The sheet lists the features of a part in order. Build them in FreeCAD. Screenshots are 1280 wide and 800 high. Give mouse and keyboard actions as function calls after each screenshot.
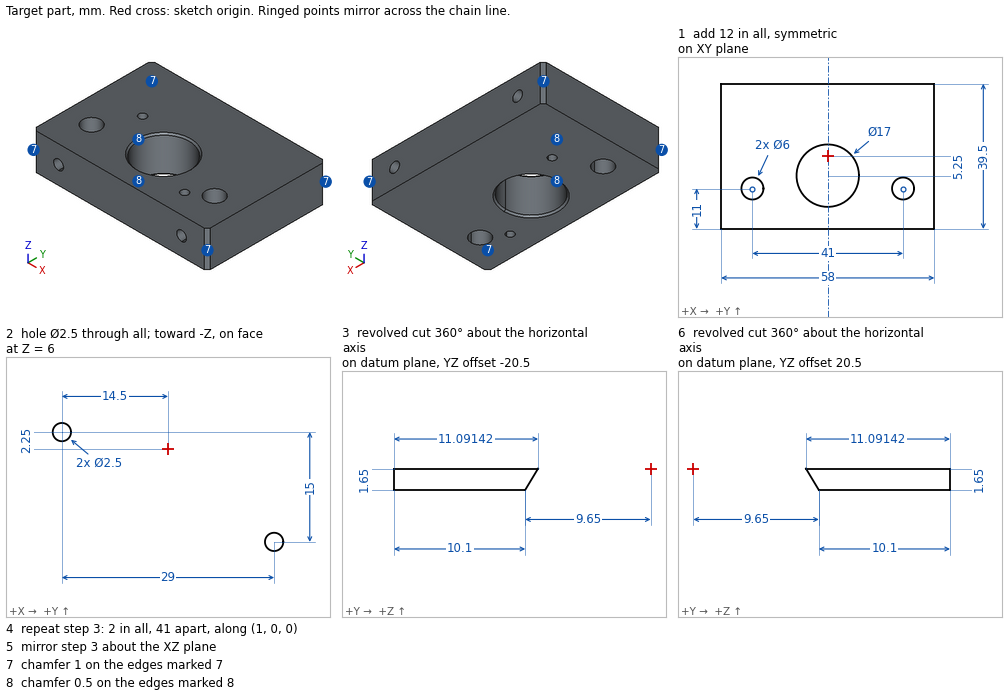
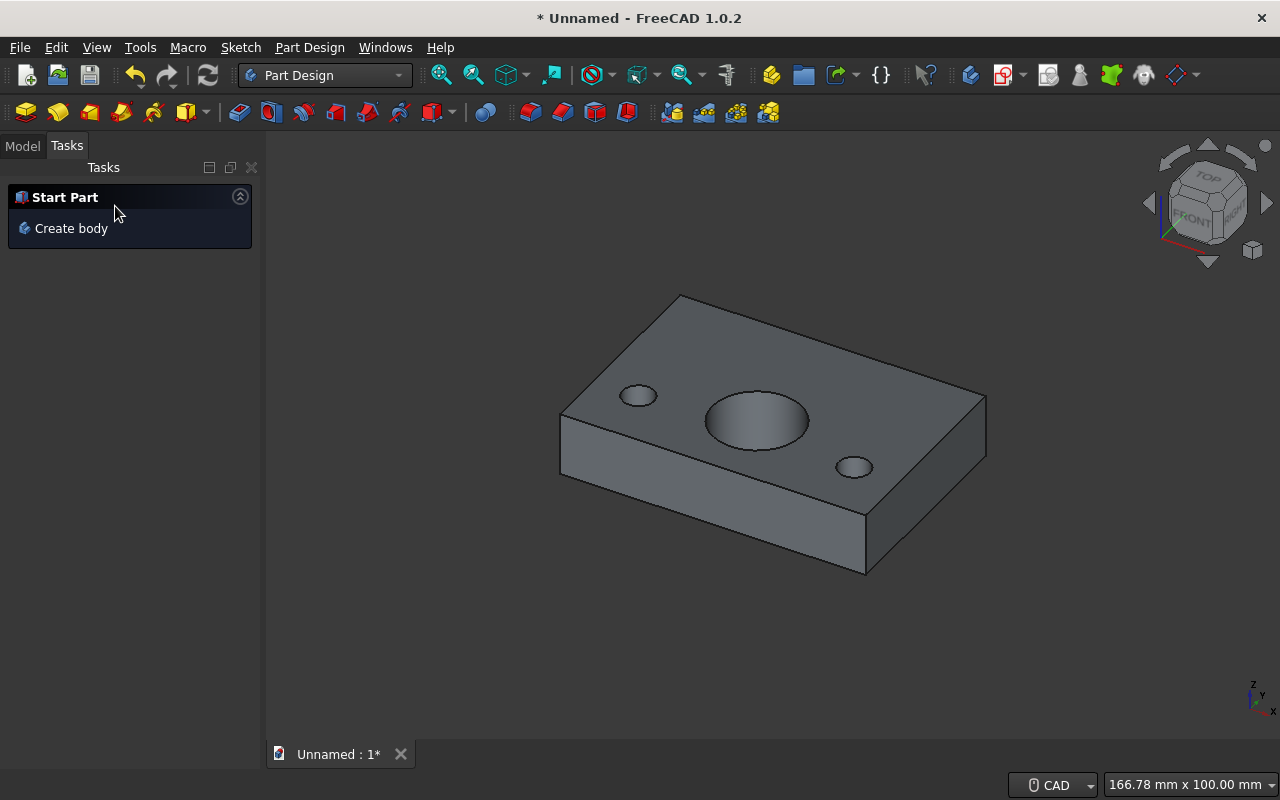
click(877, 416)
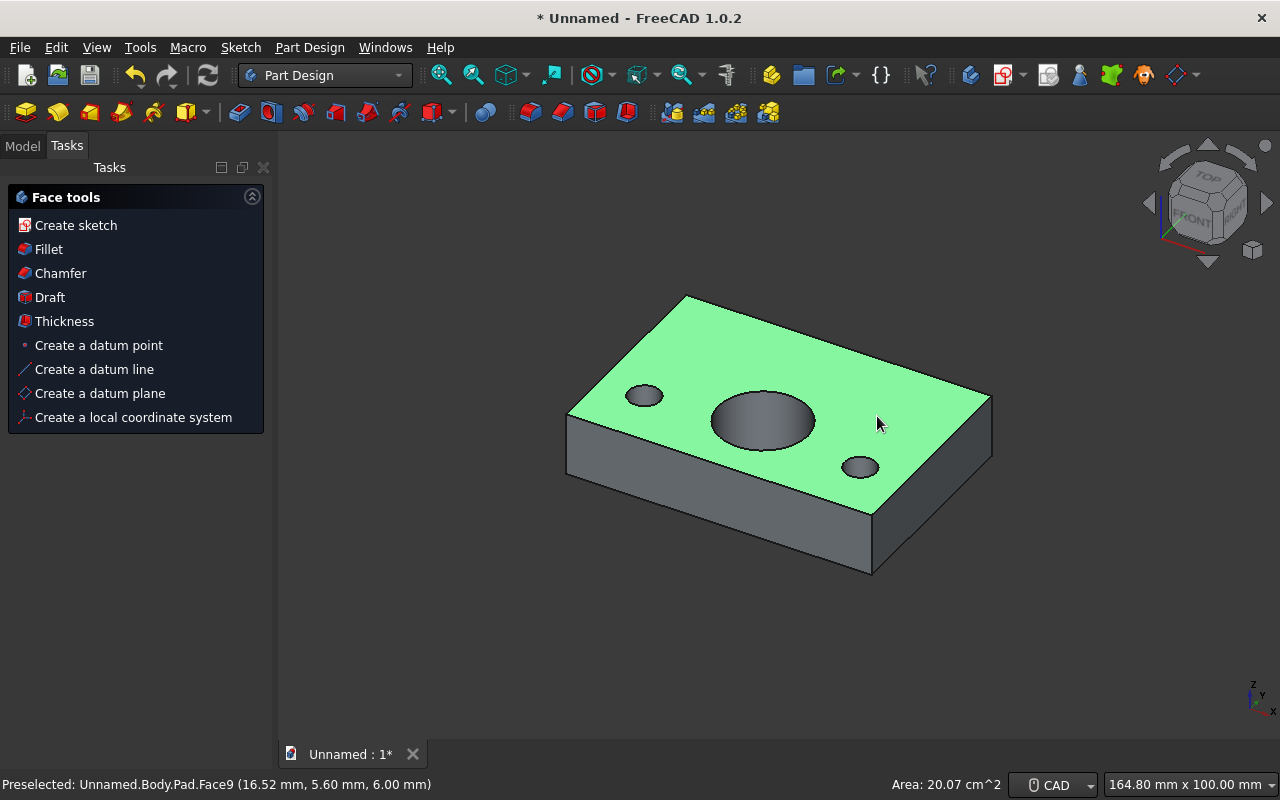
click(1004, 76)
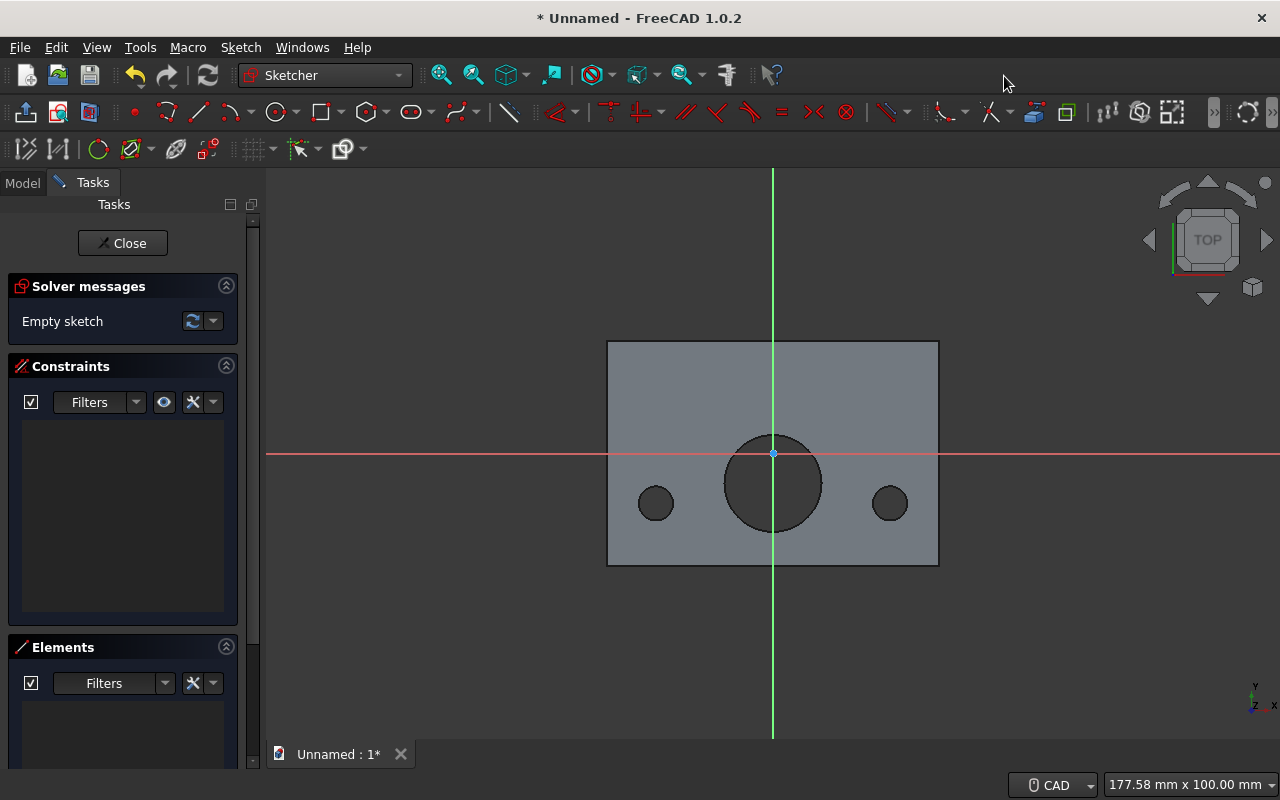
scroll(803, 496, up, 6)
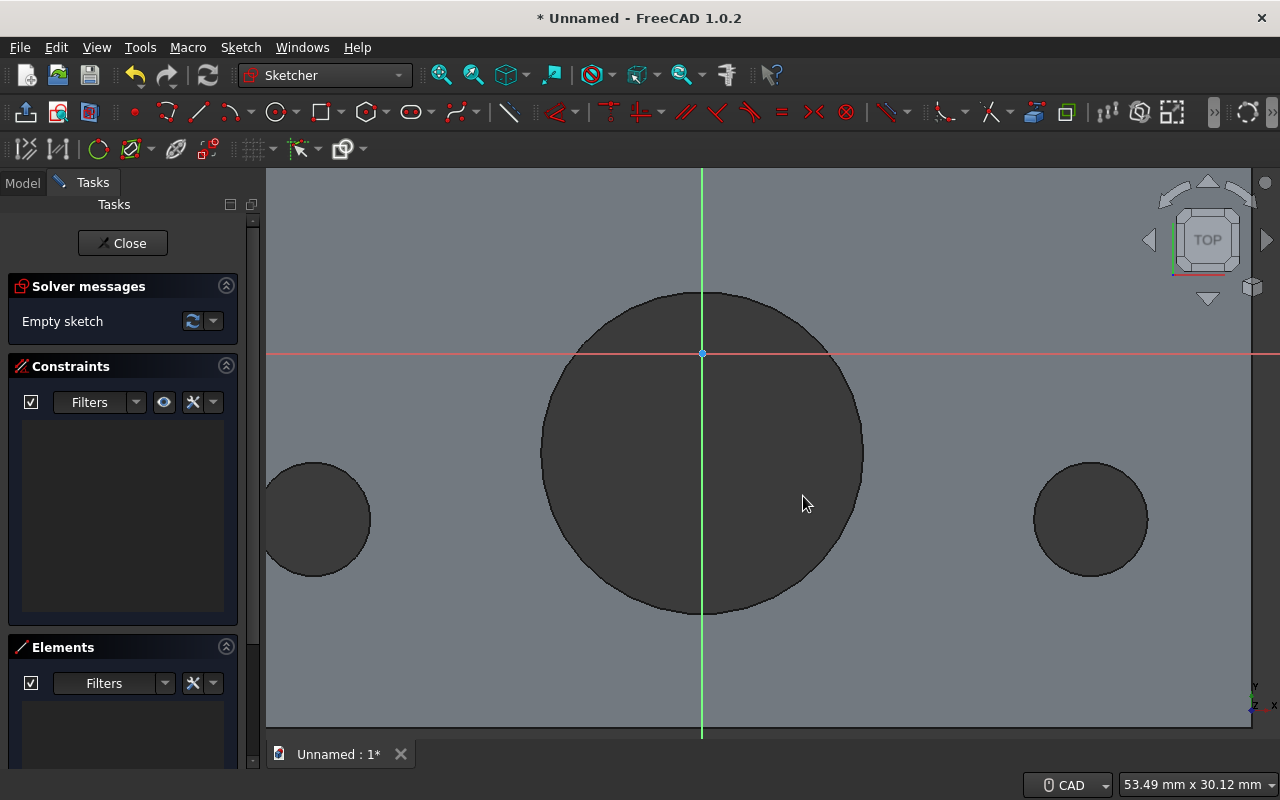
click(276, 112)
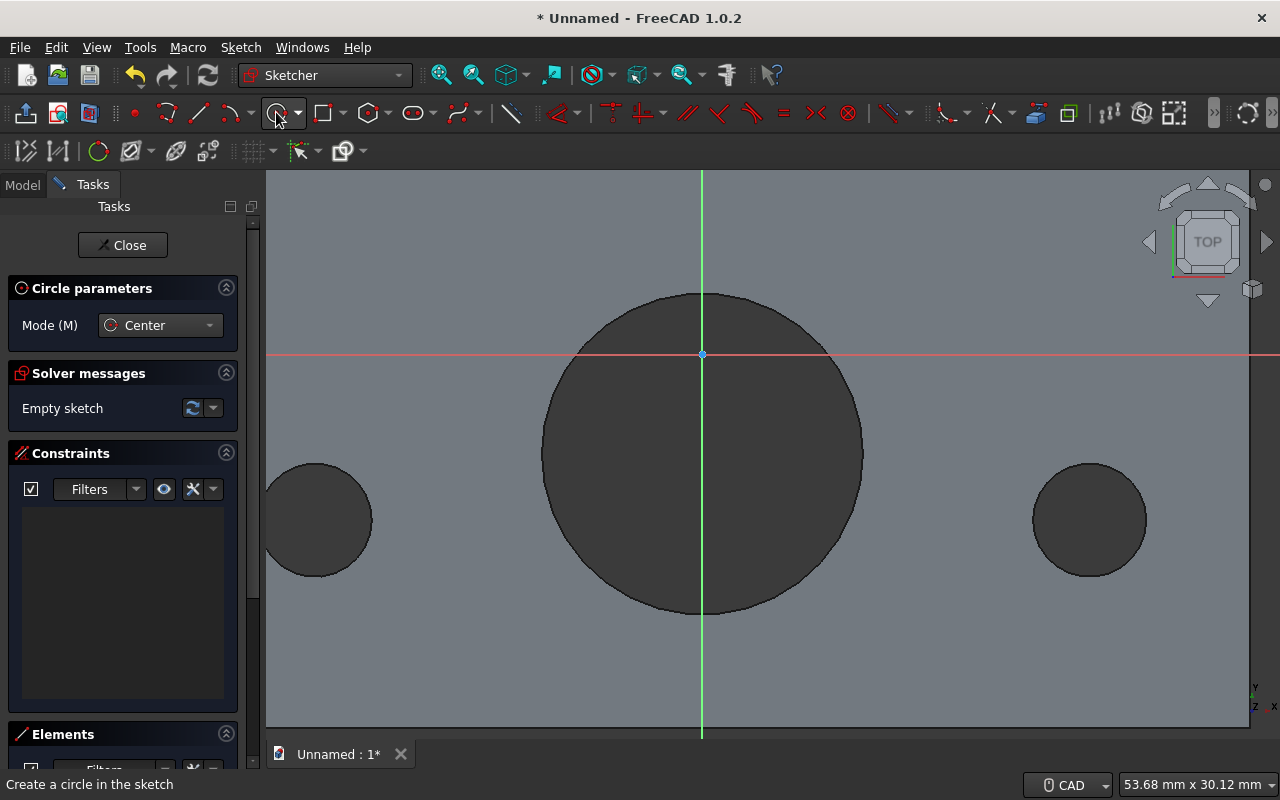
click(428, 312)
click(445, 296)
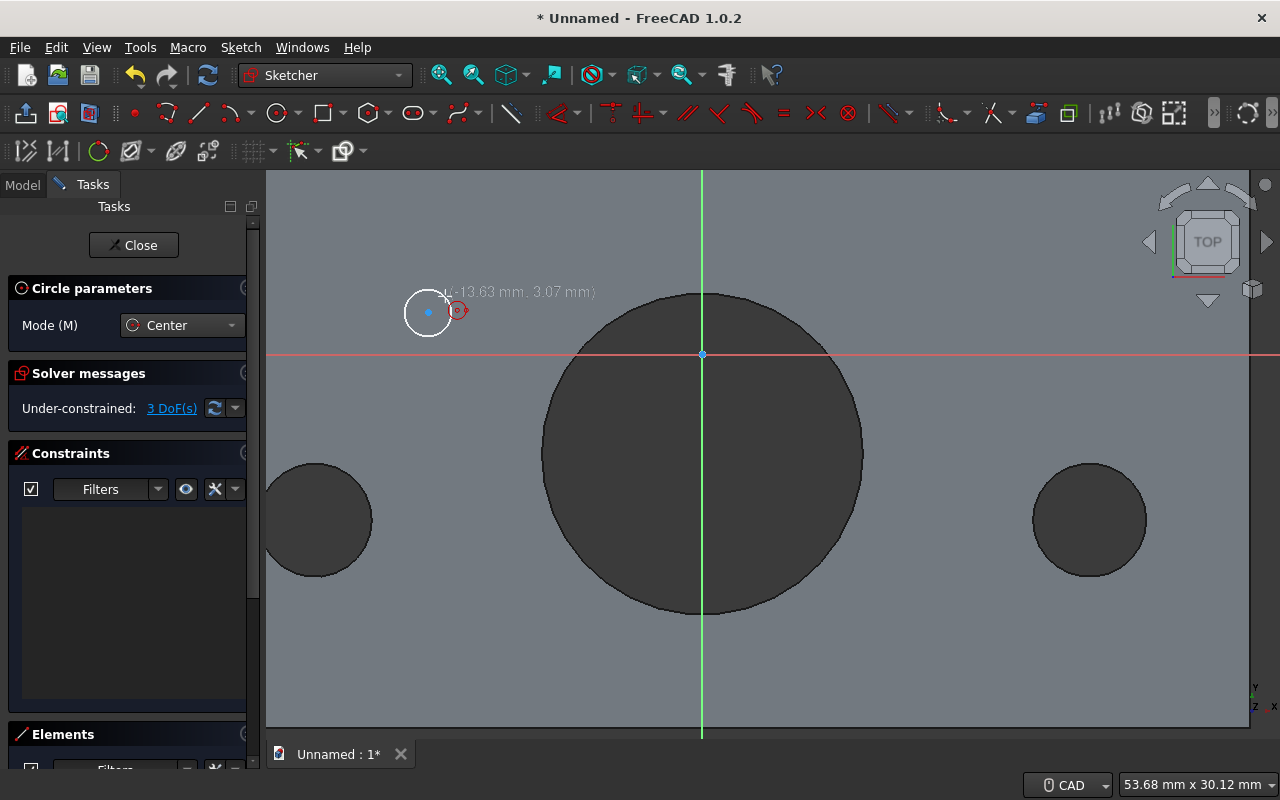
click(976, 596)
click(993, 579)
key(Escape)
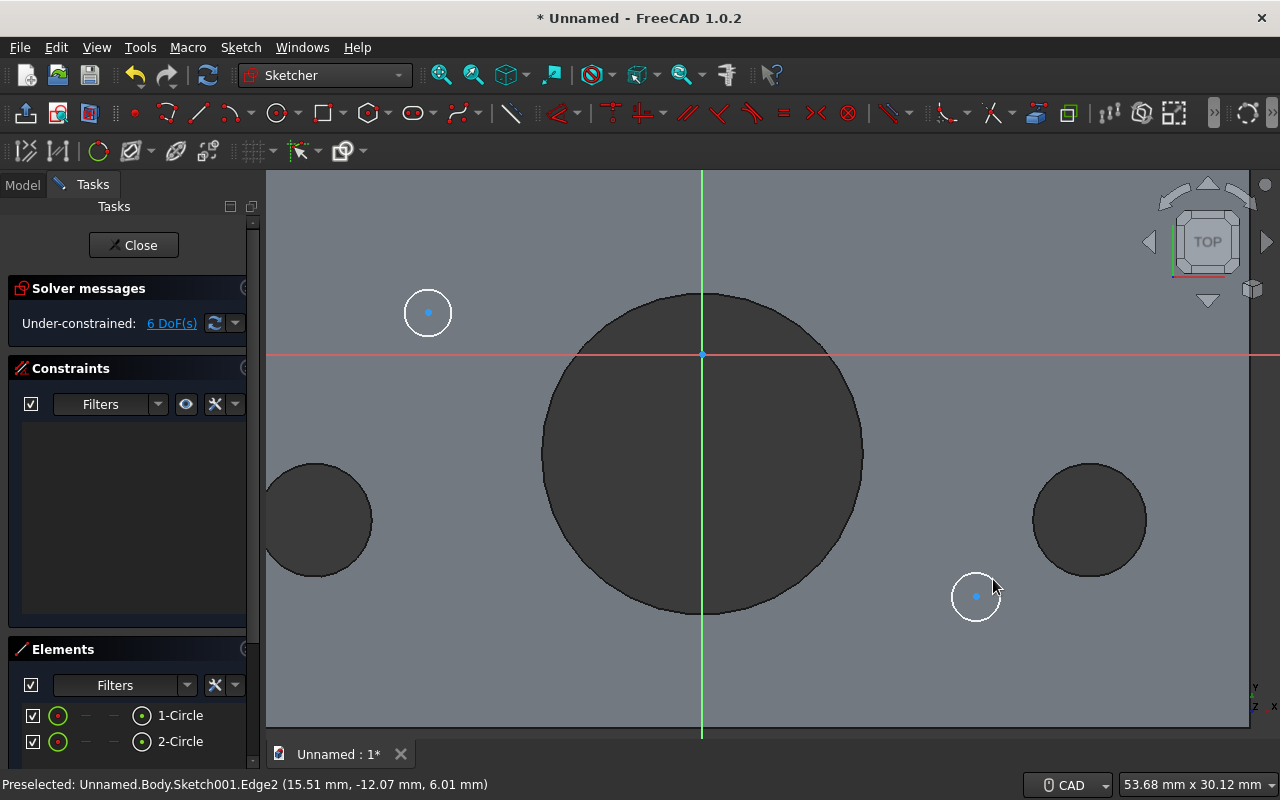
click(444, 296)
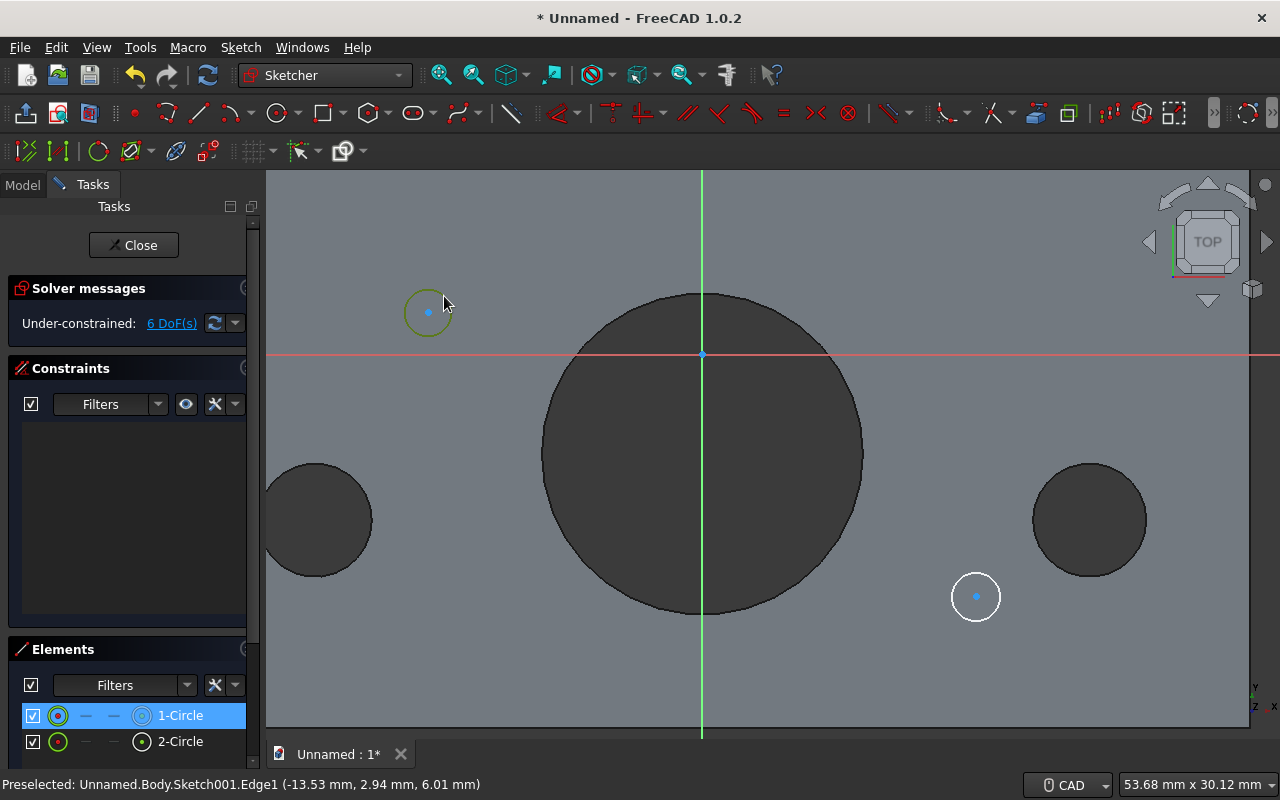
click(993, 580)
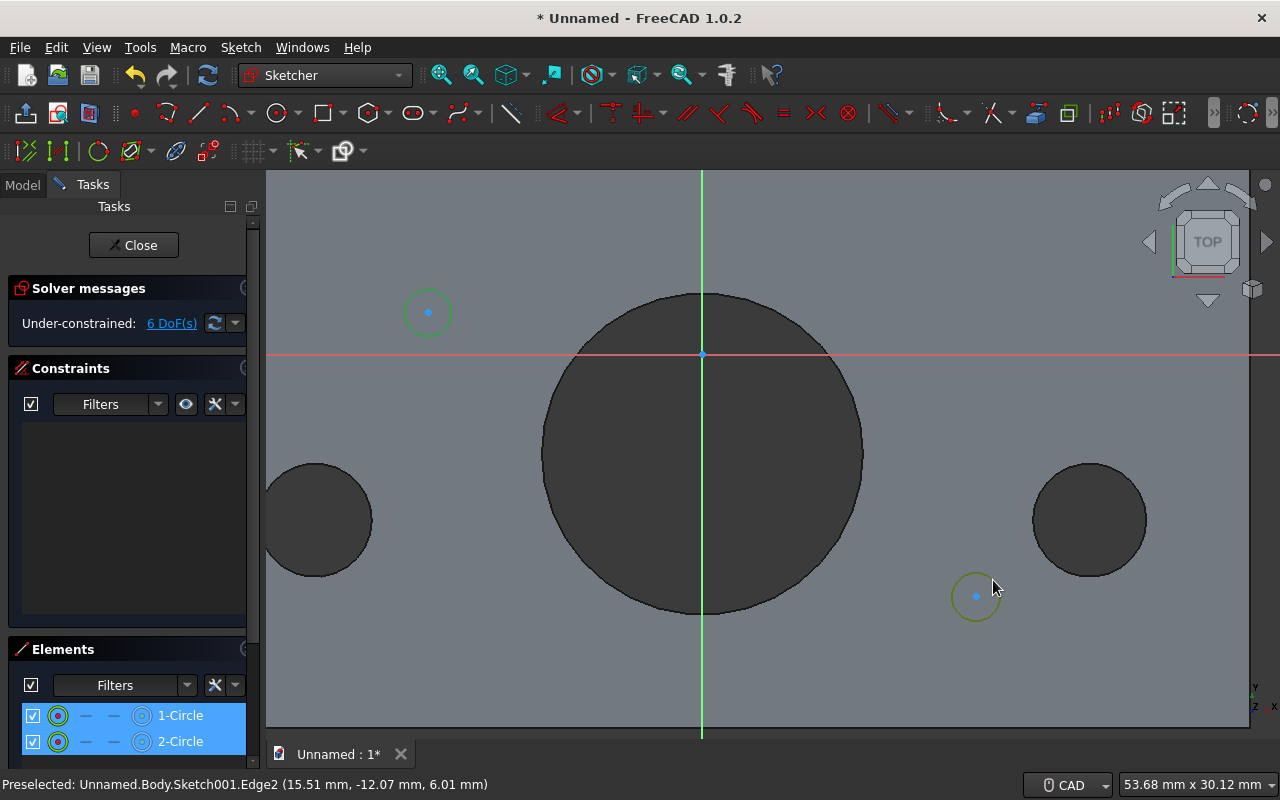
key(e)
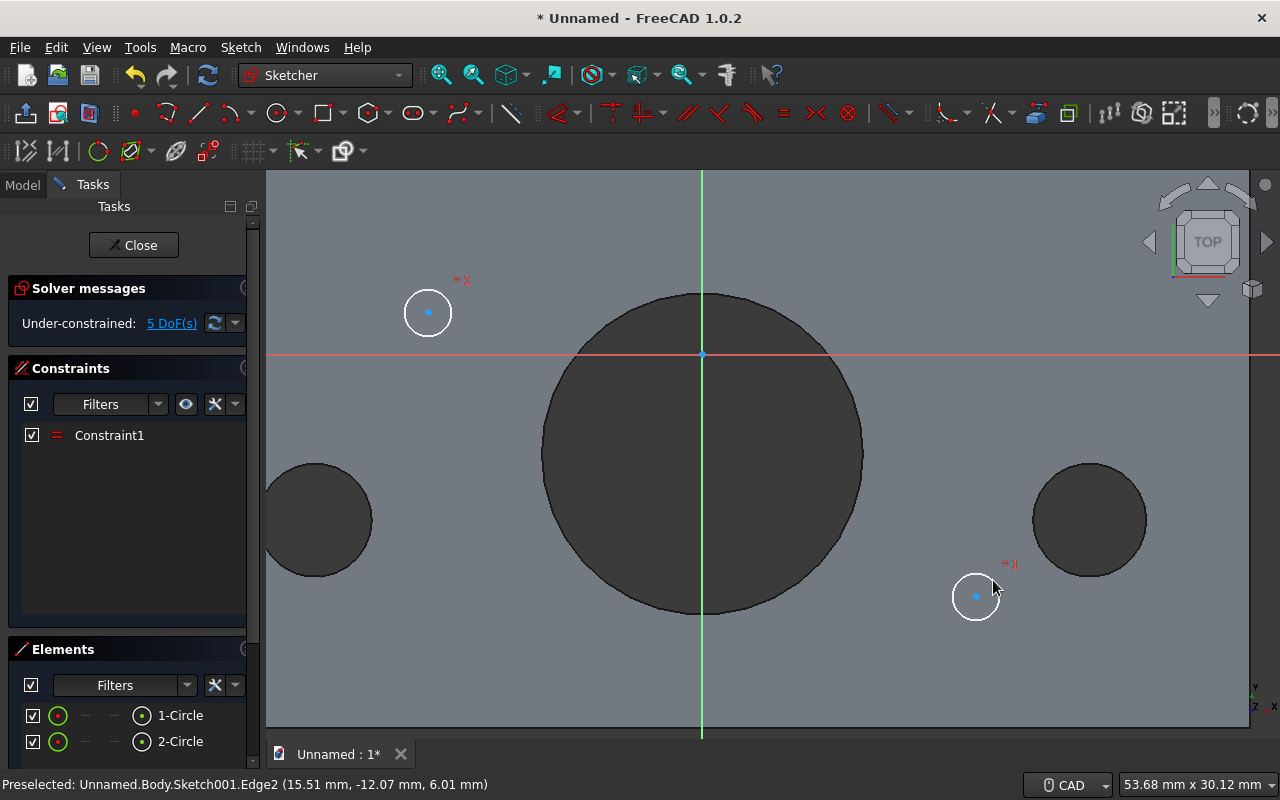
key(d)